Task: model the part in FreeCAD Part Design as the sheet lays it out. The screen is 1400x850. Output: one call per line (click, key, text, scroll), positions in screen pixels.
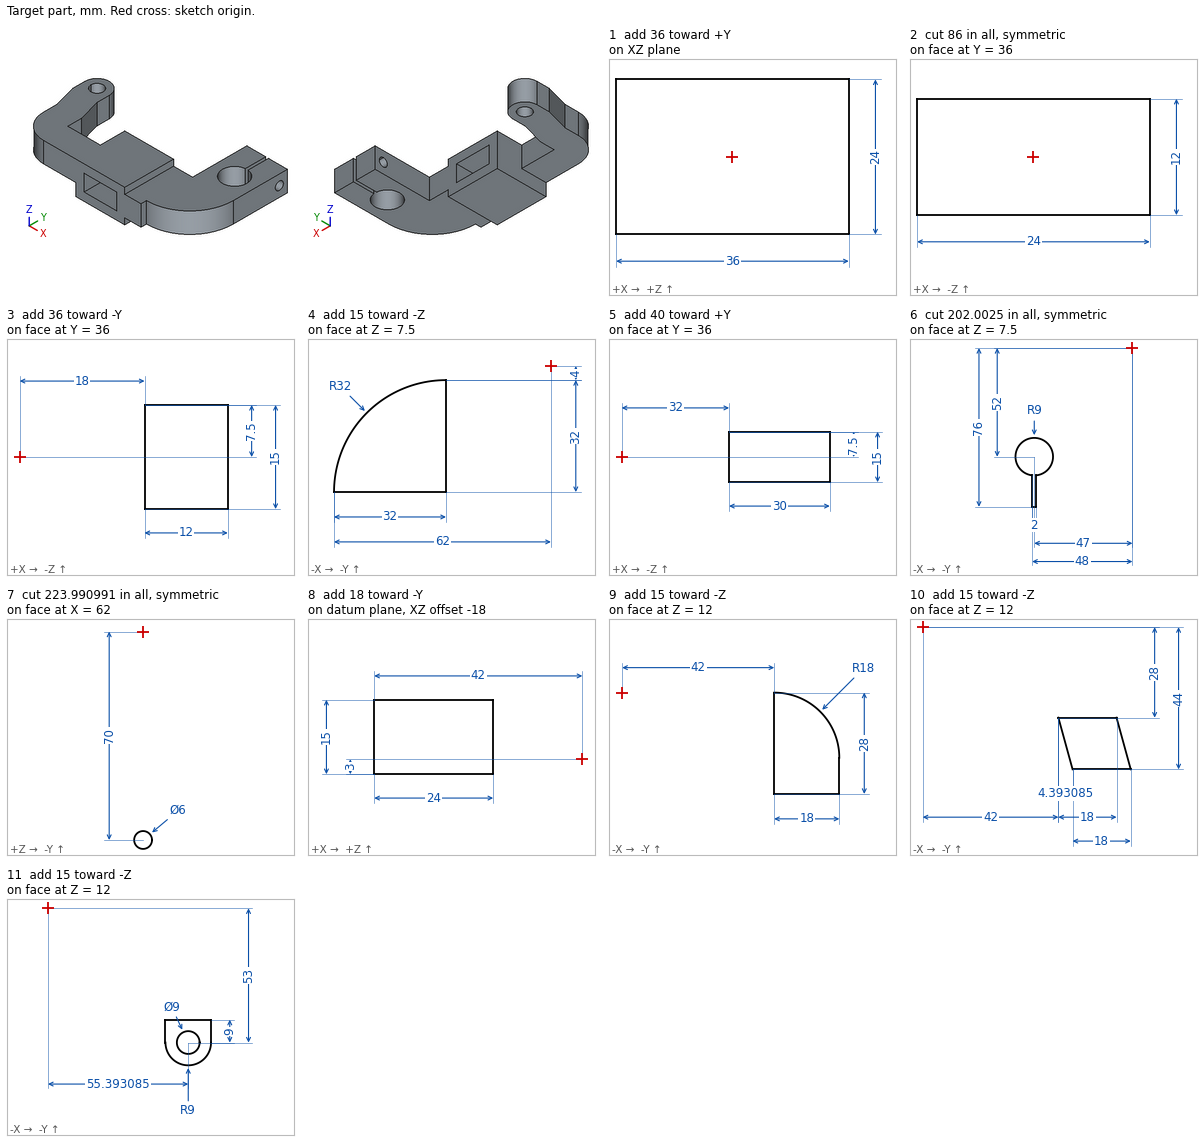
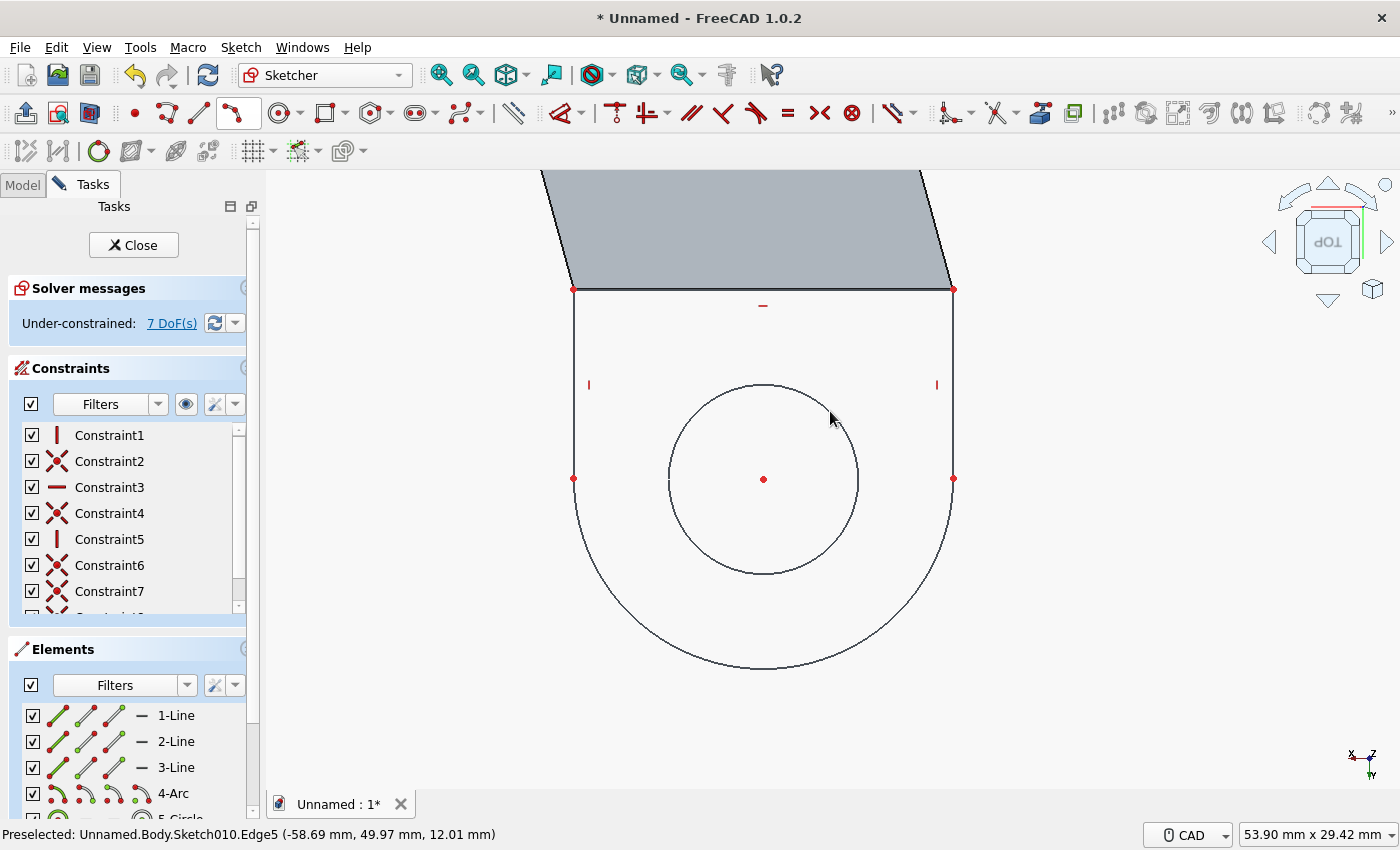
click(953, 422)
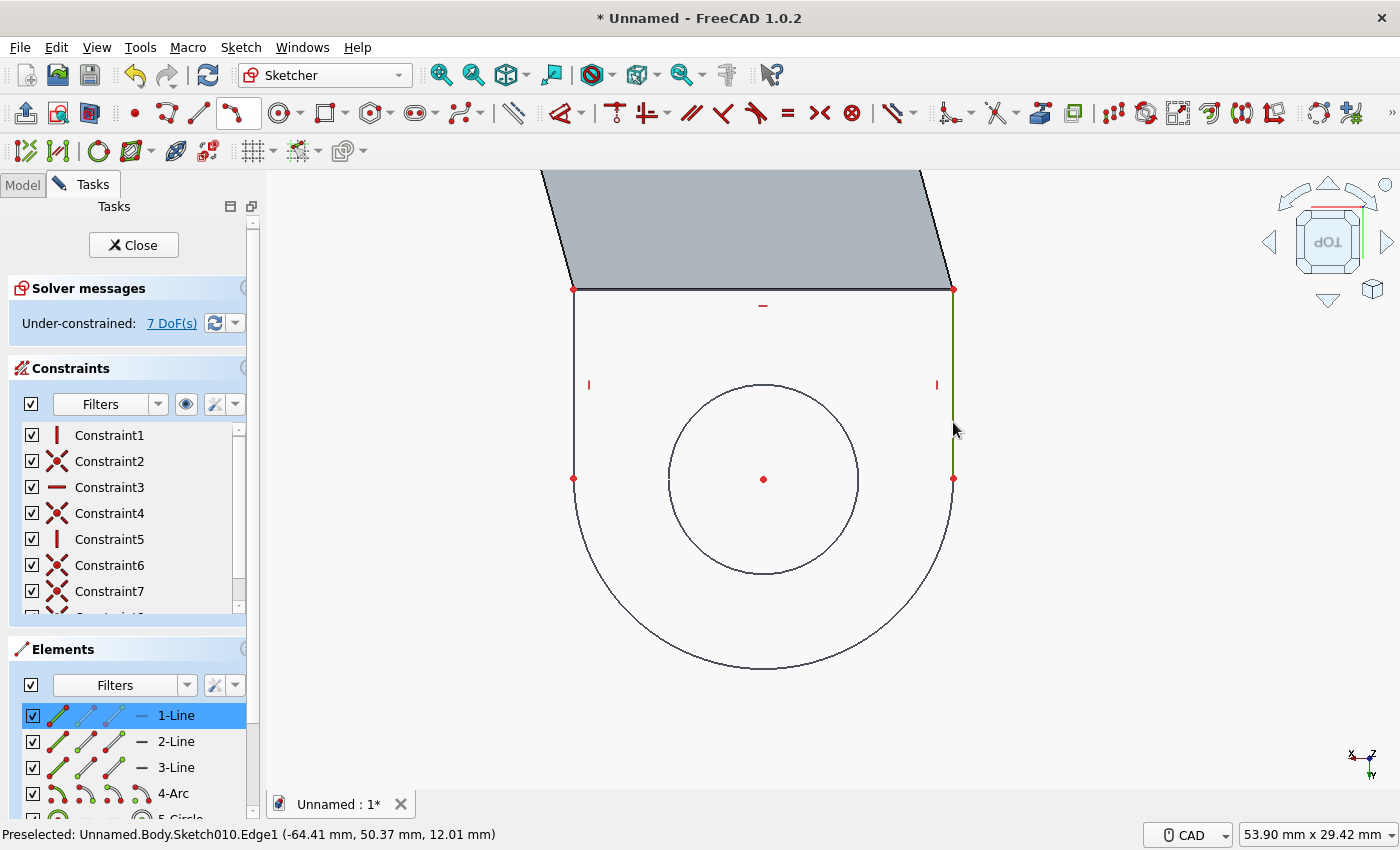
click(652, 633)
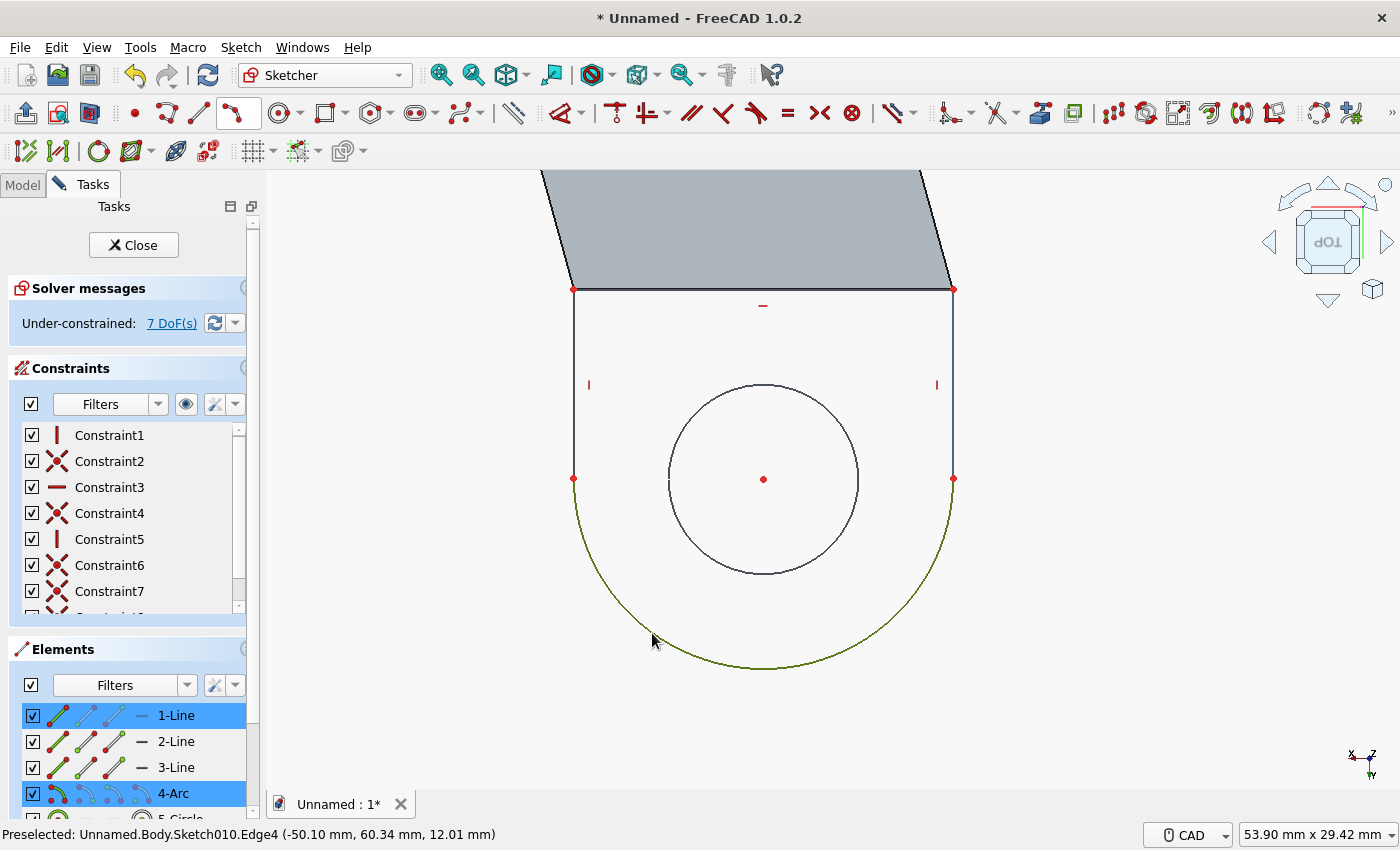
key(t)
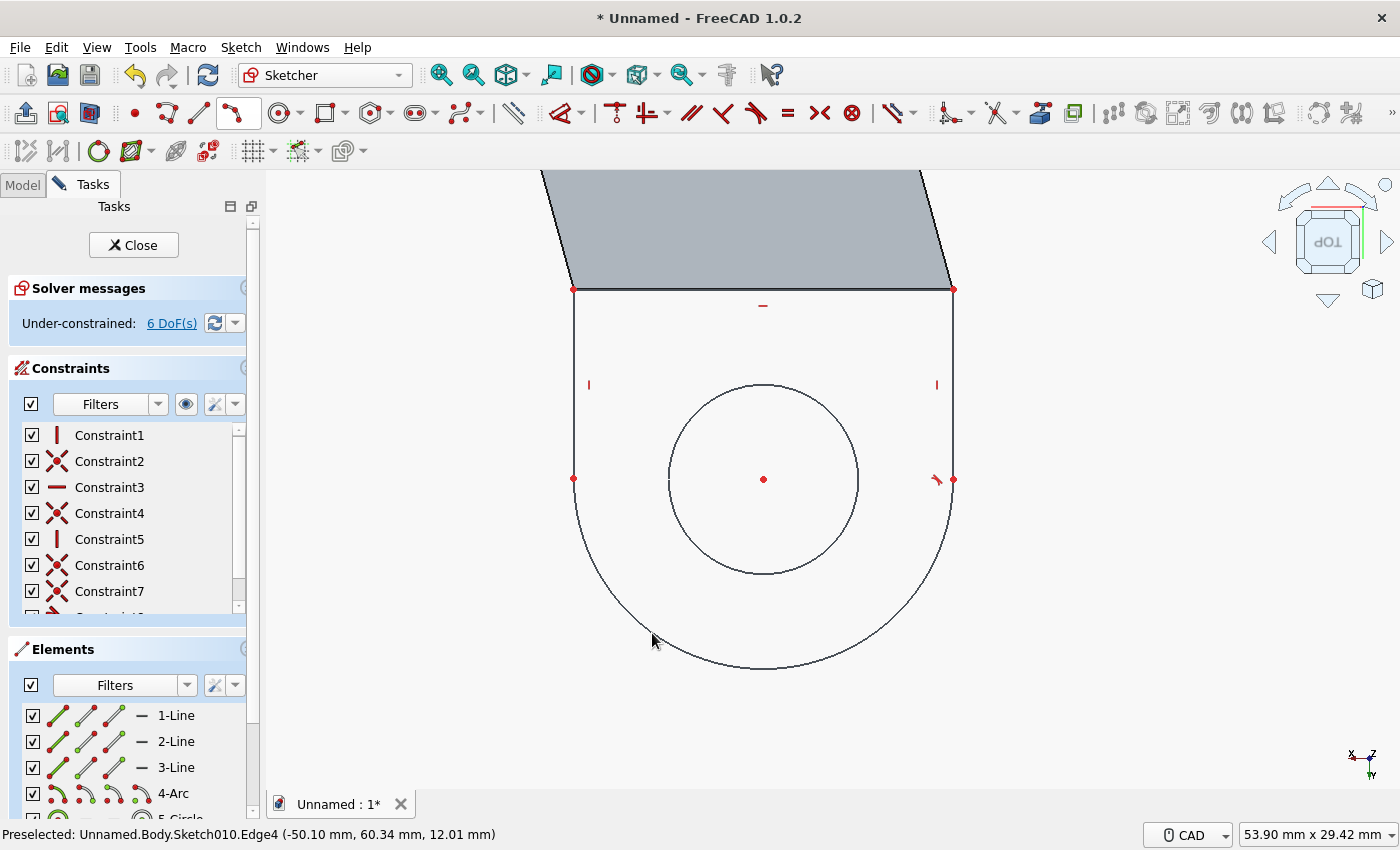
click(574, 347)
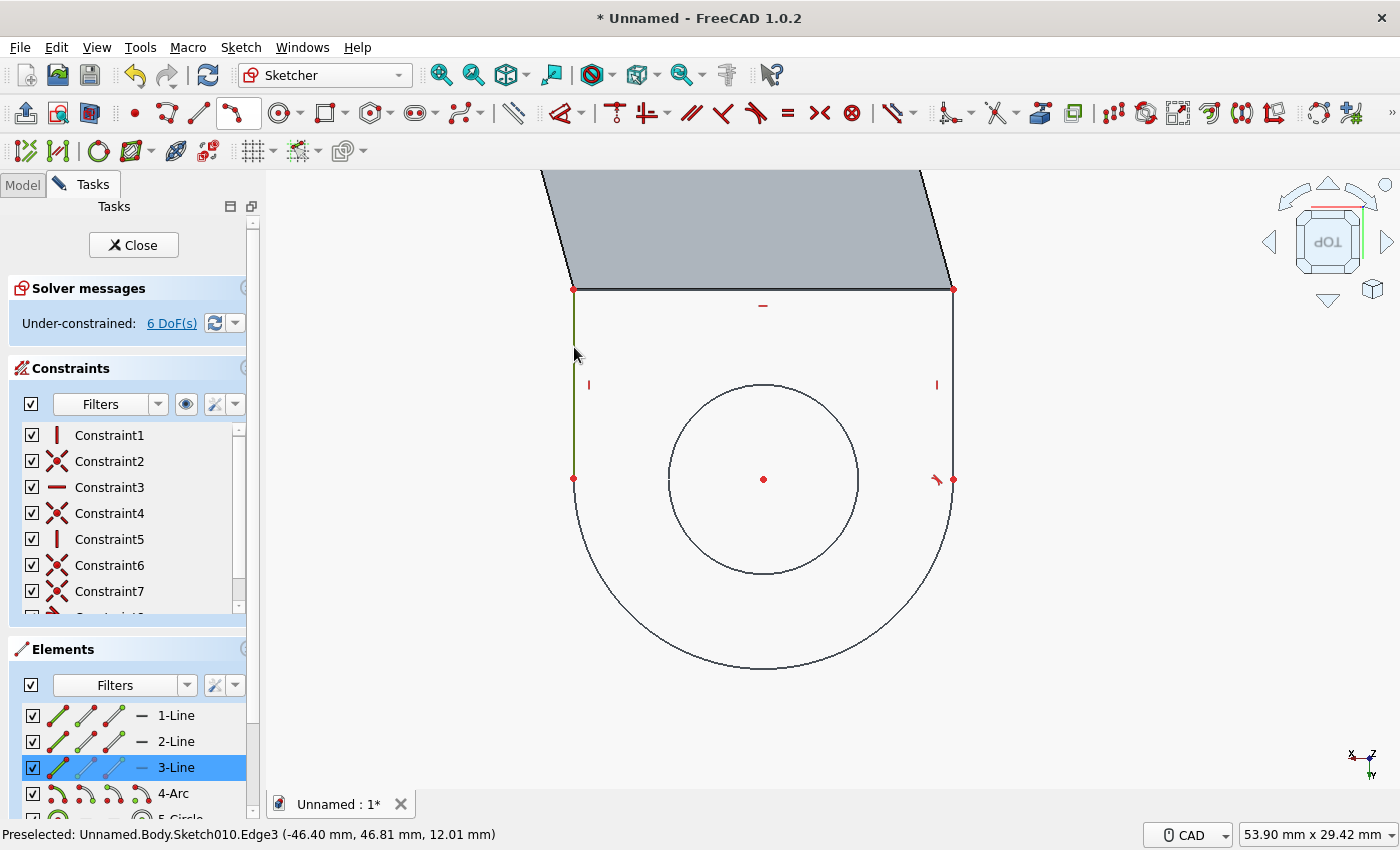
click(652, 633)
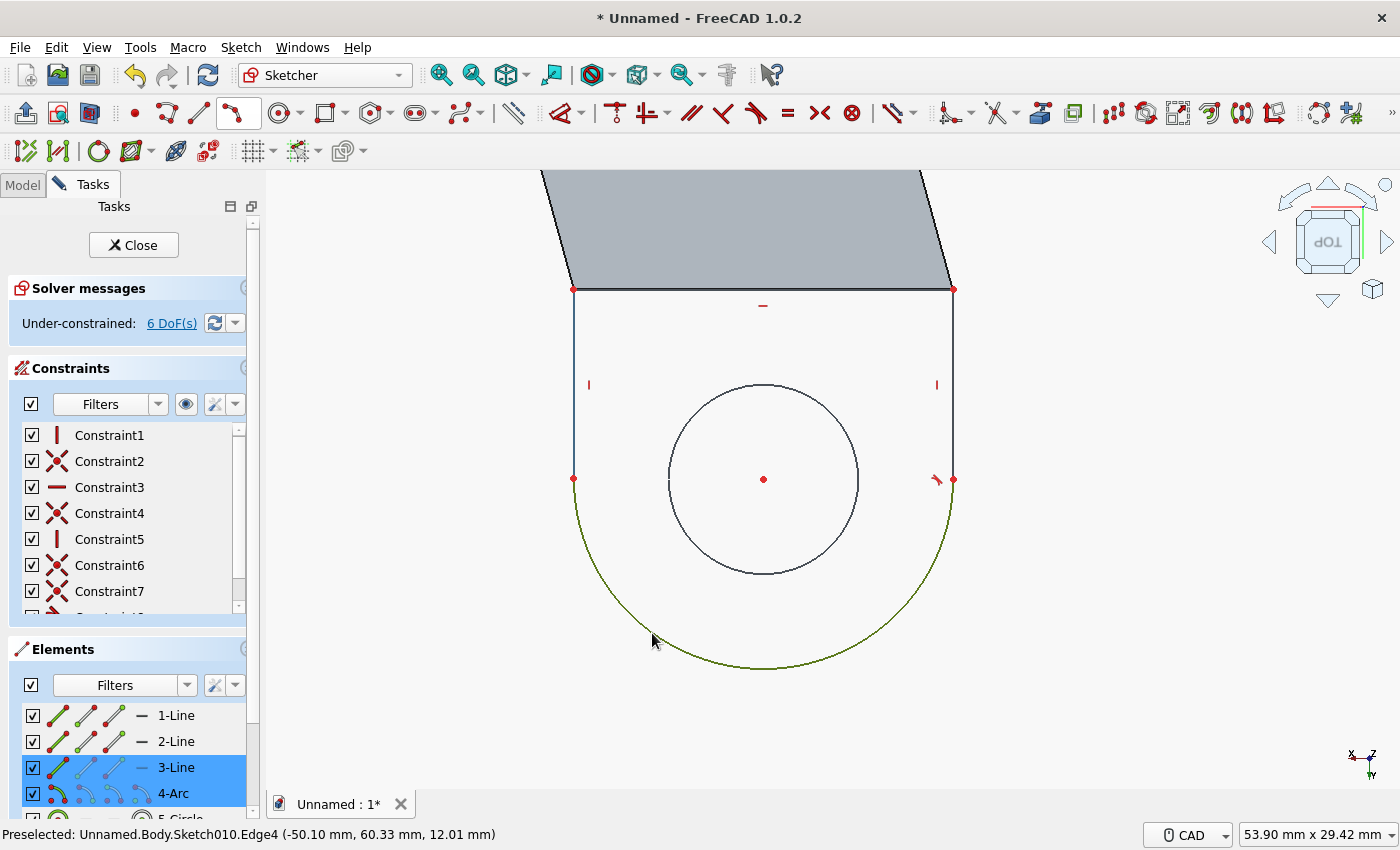
key(t)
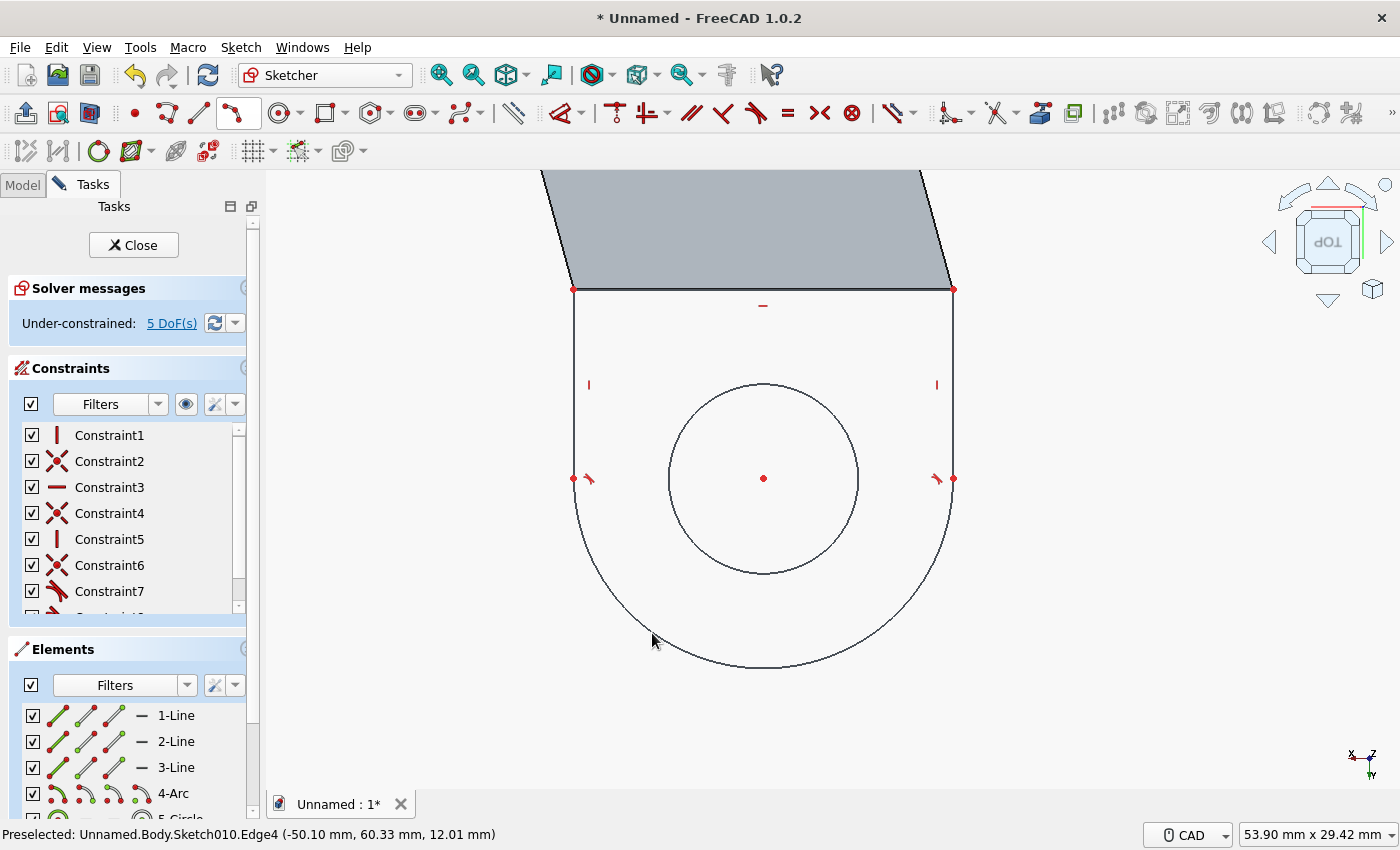
key(d)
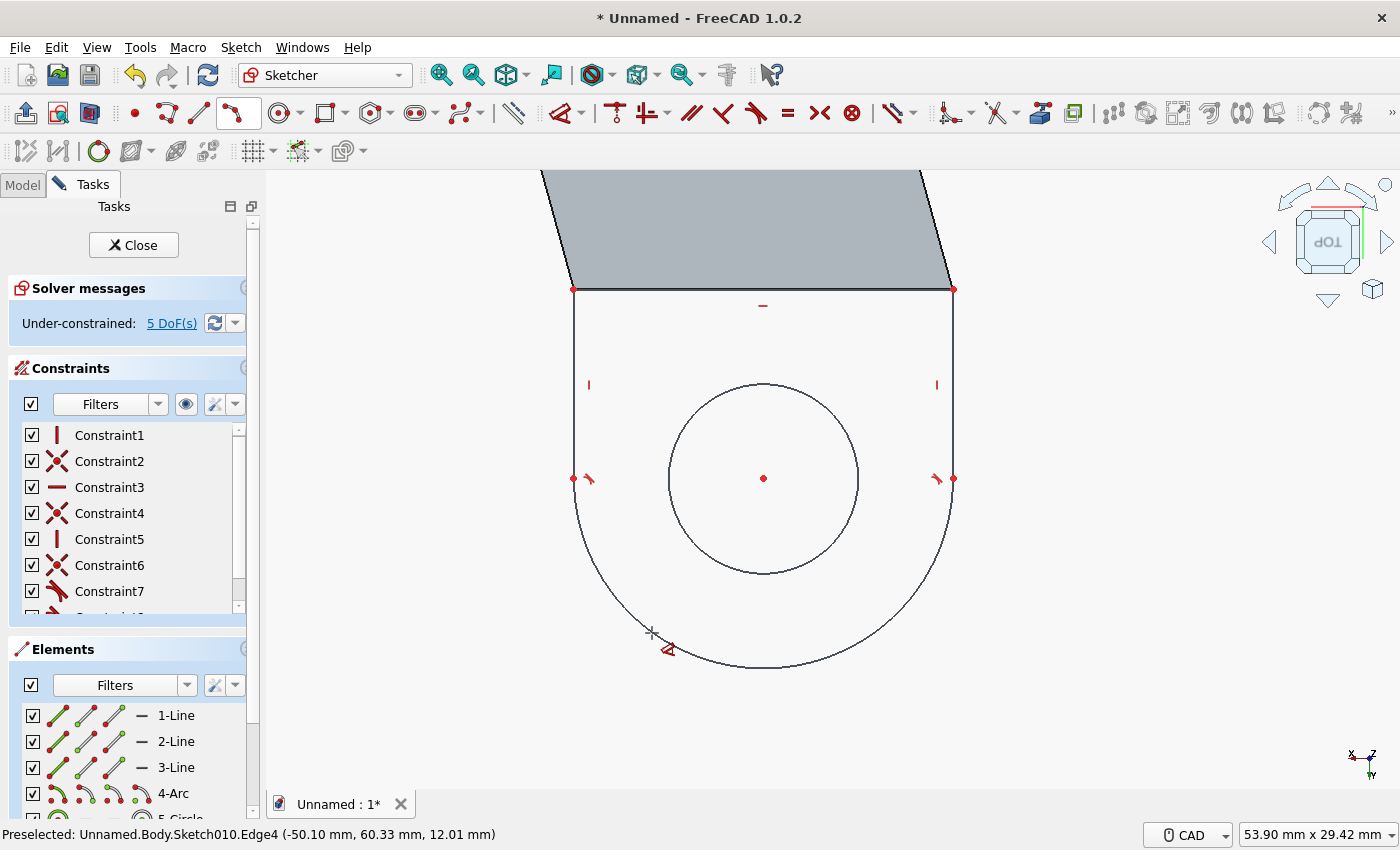
click(652, 632)
click(633, 658)